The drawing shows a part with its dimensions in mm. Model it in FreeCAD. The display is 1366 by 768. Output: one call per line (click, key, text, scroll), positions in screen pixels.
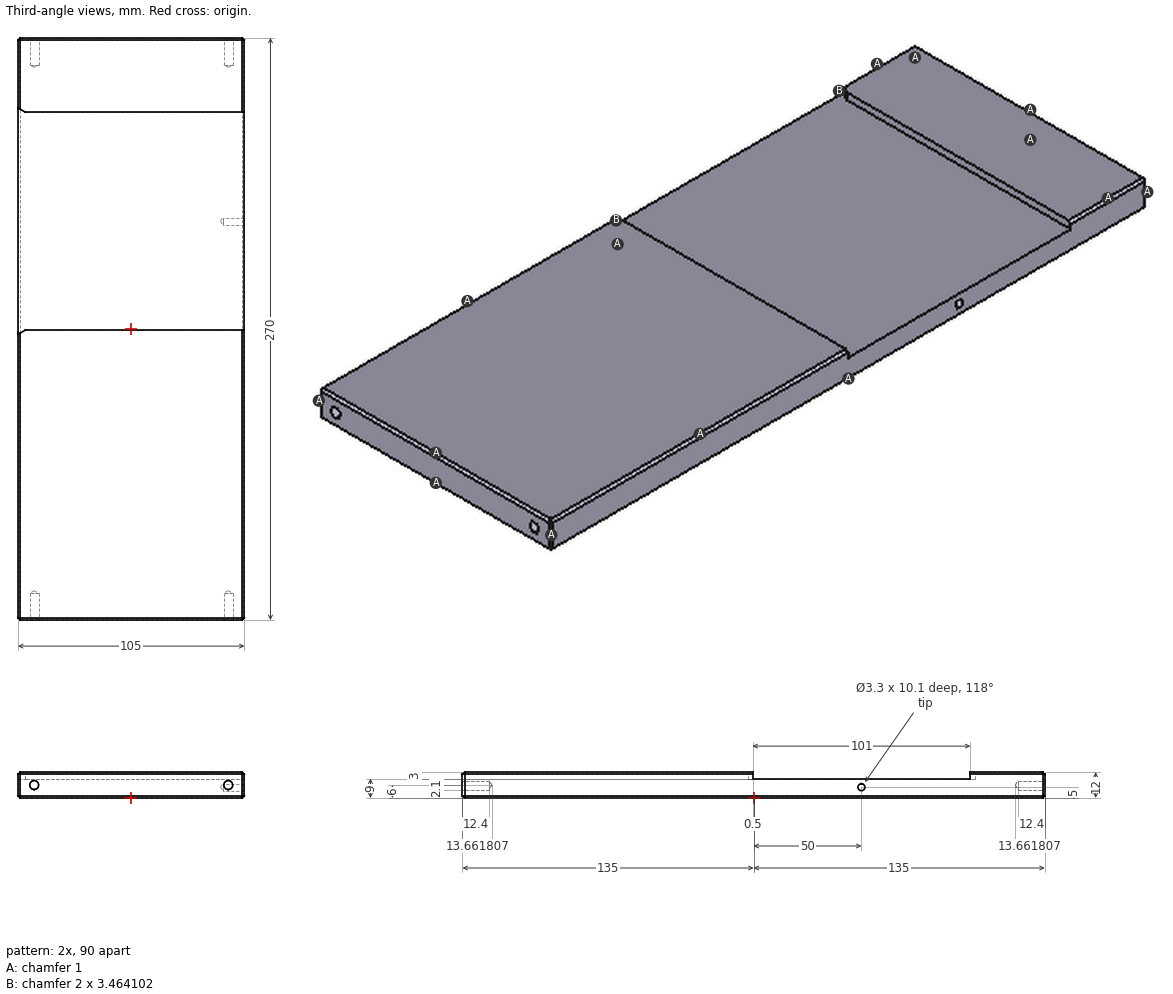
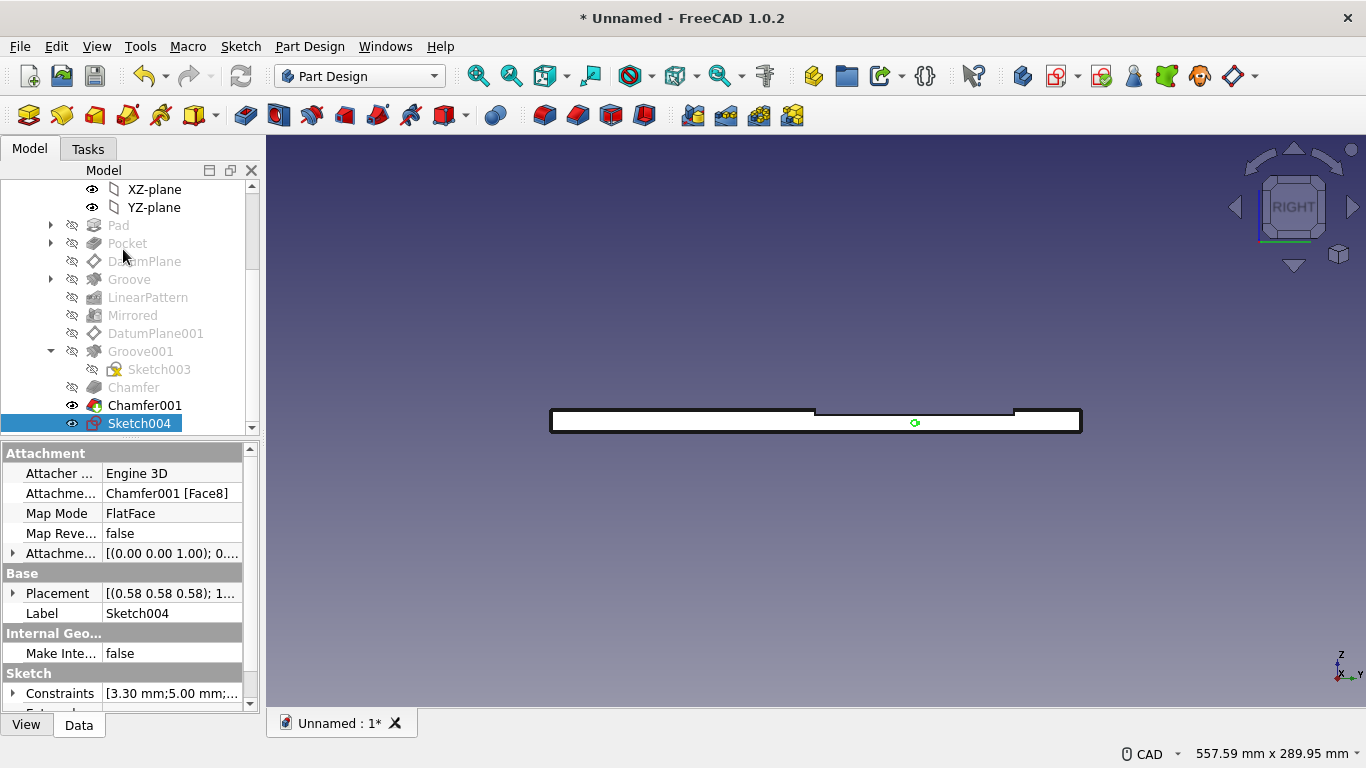
click(279, 116)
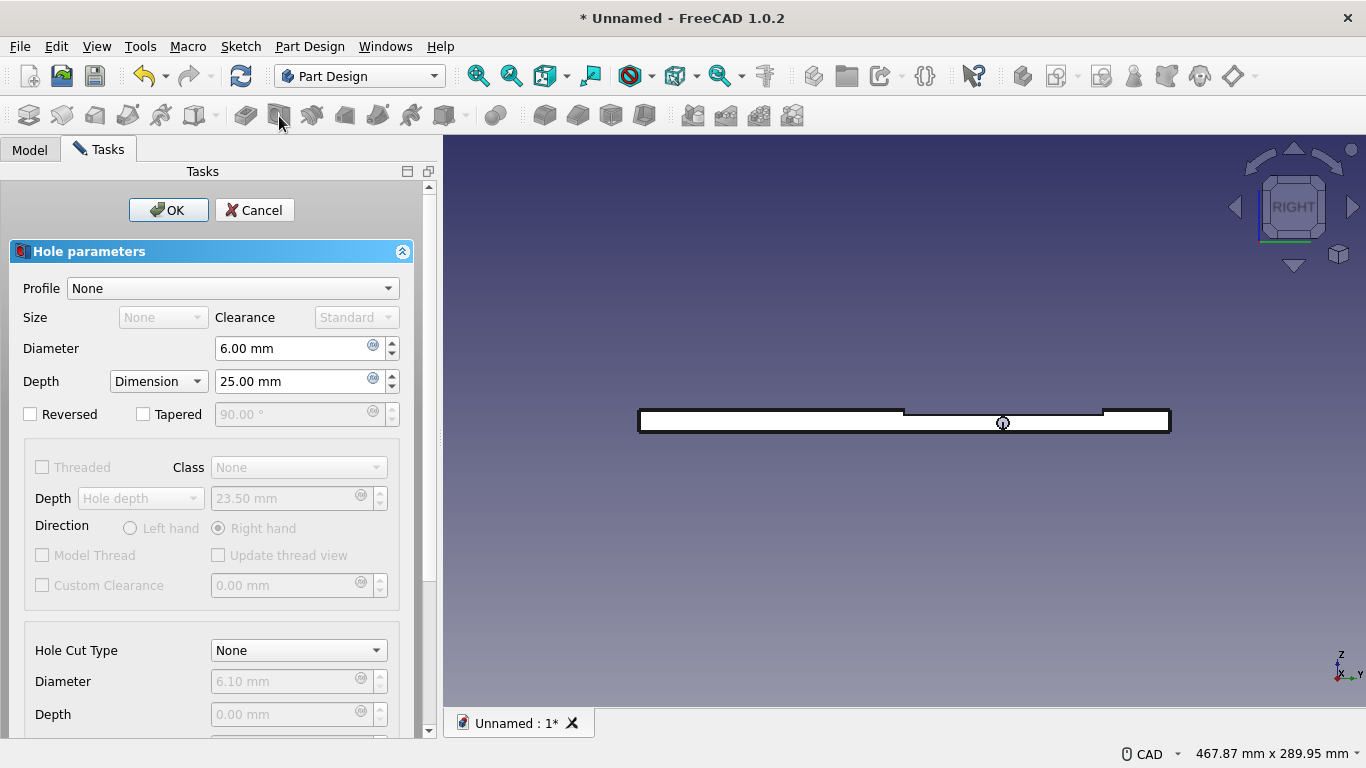
triple_click(300, 348)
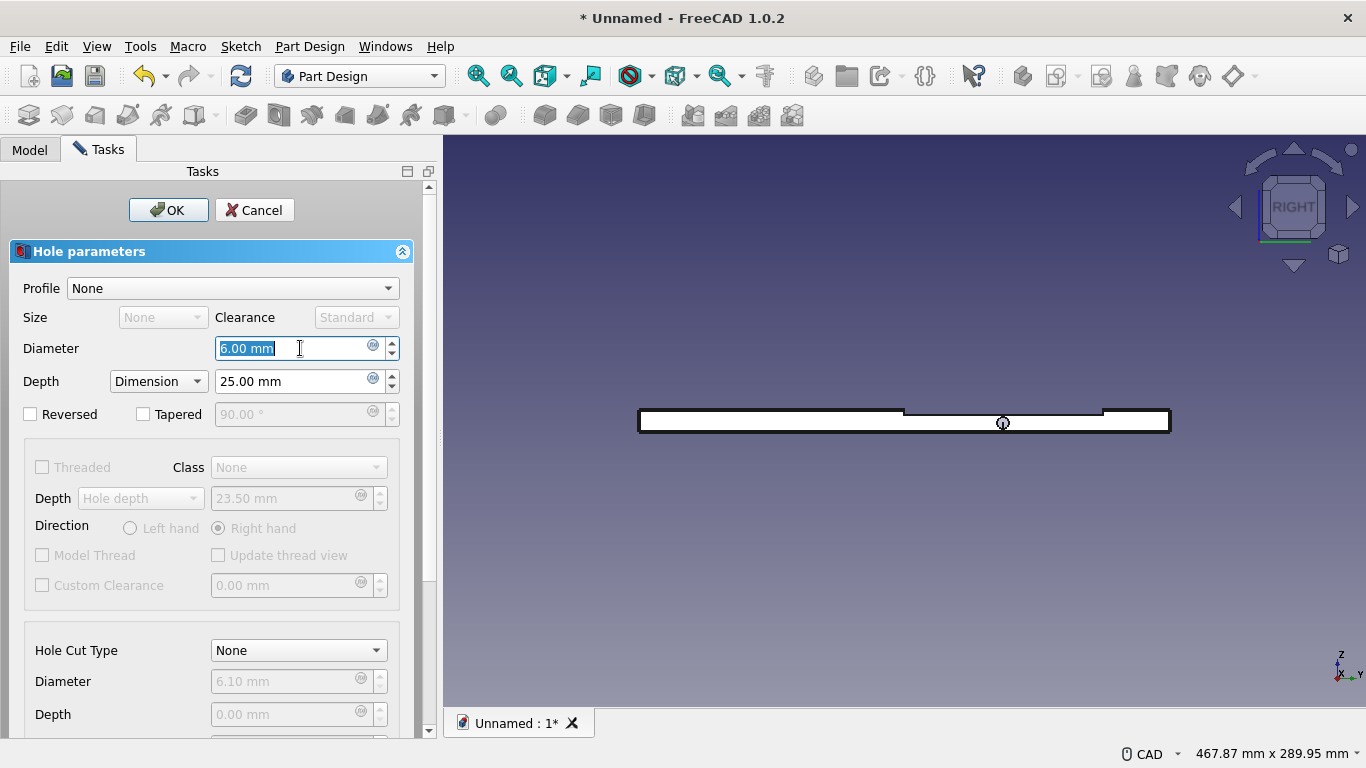
text(3.3)
key(Tab)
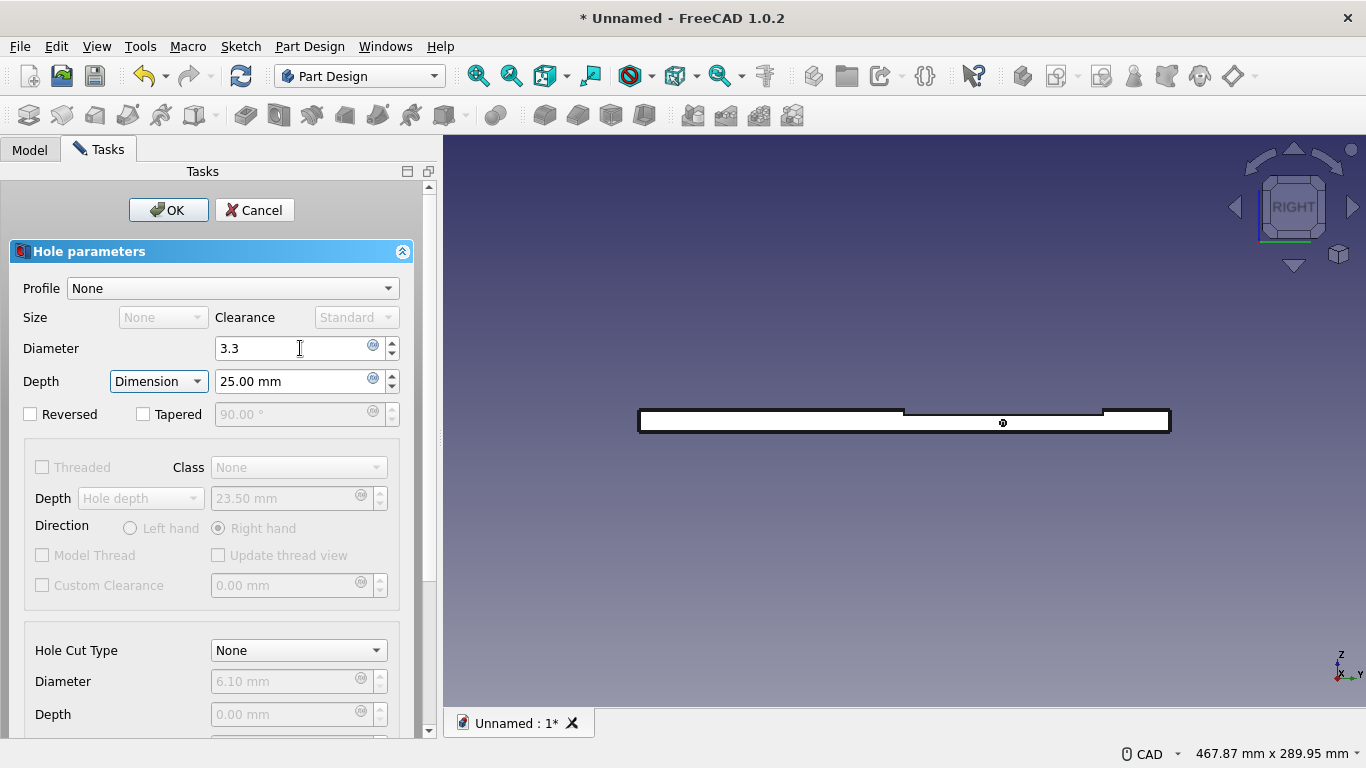
triple_click(300, 382)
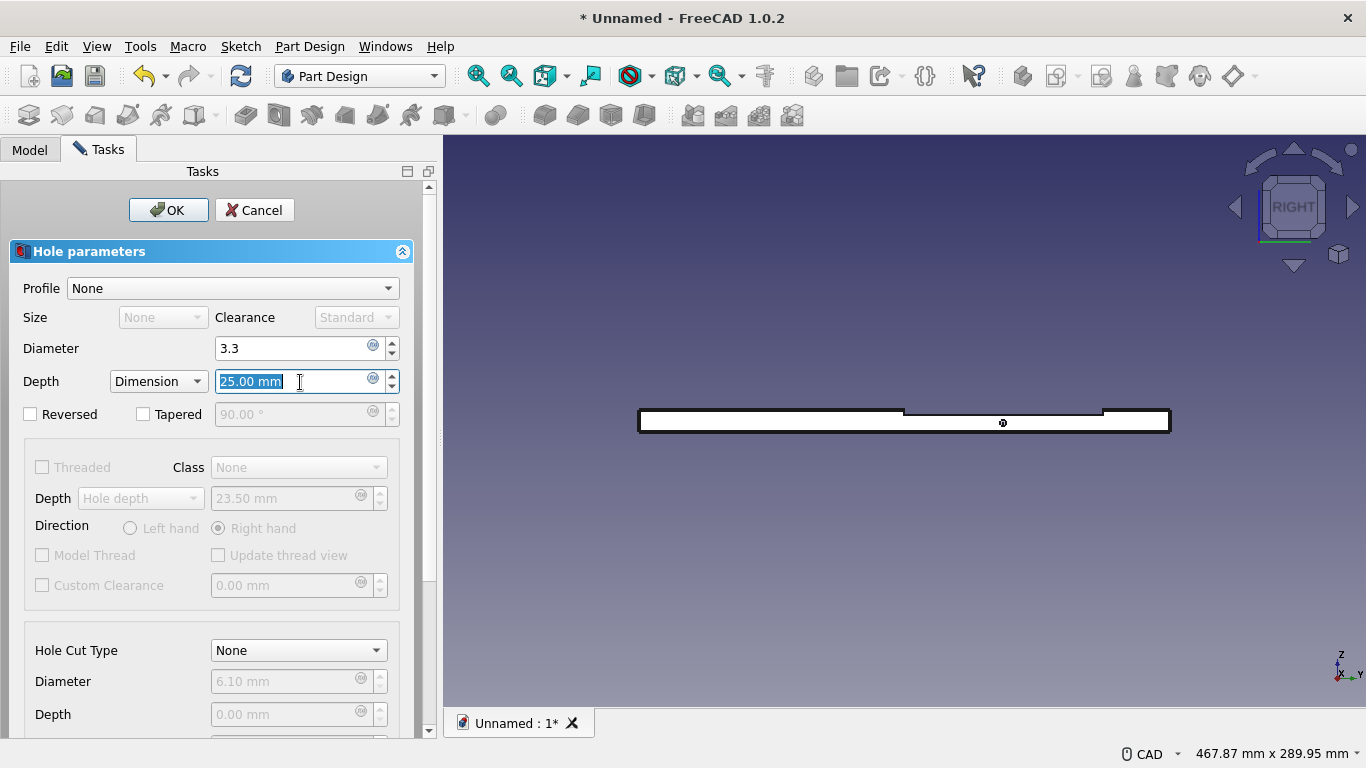
text(10.1)
key(Tab)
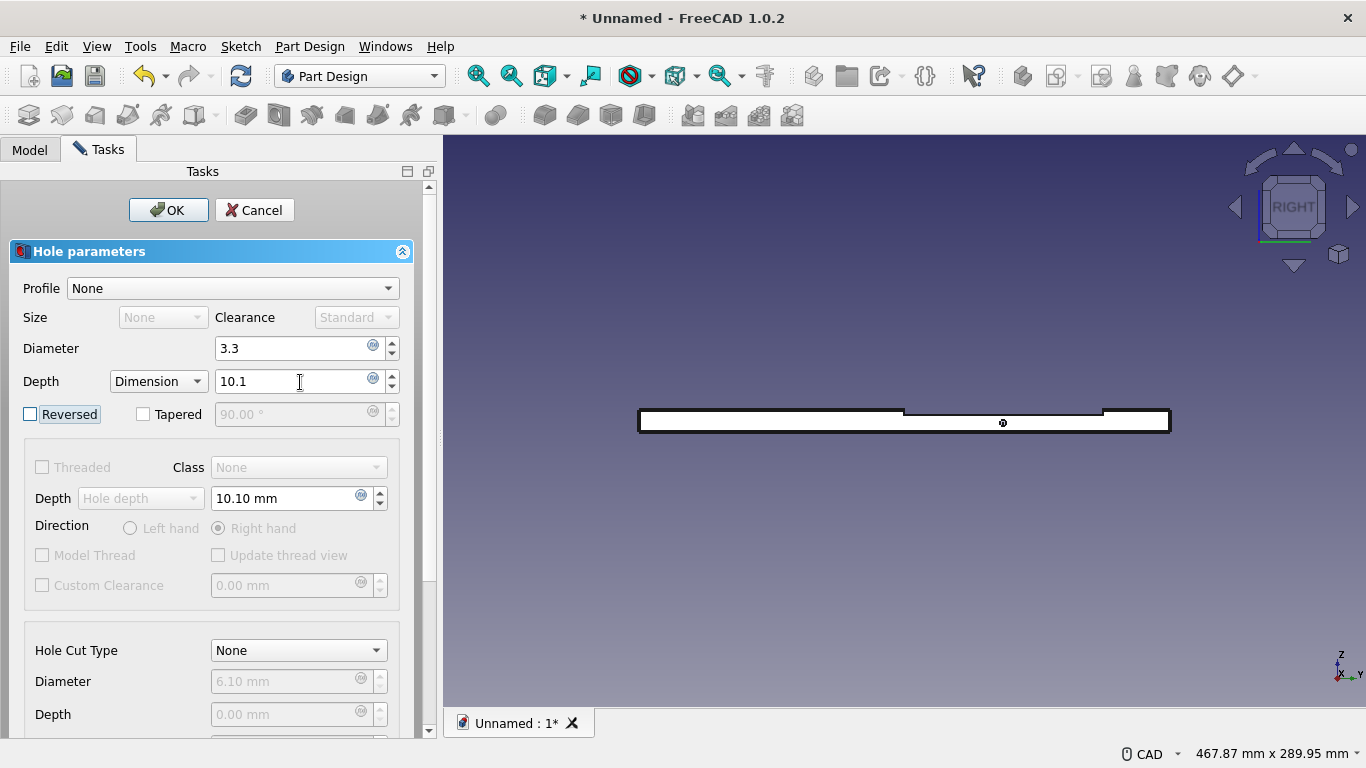
click(169, 210)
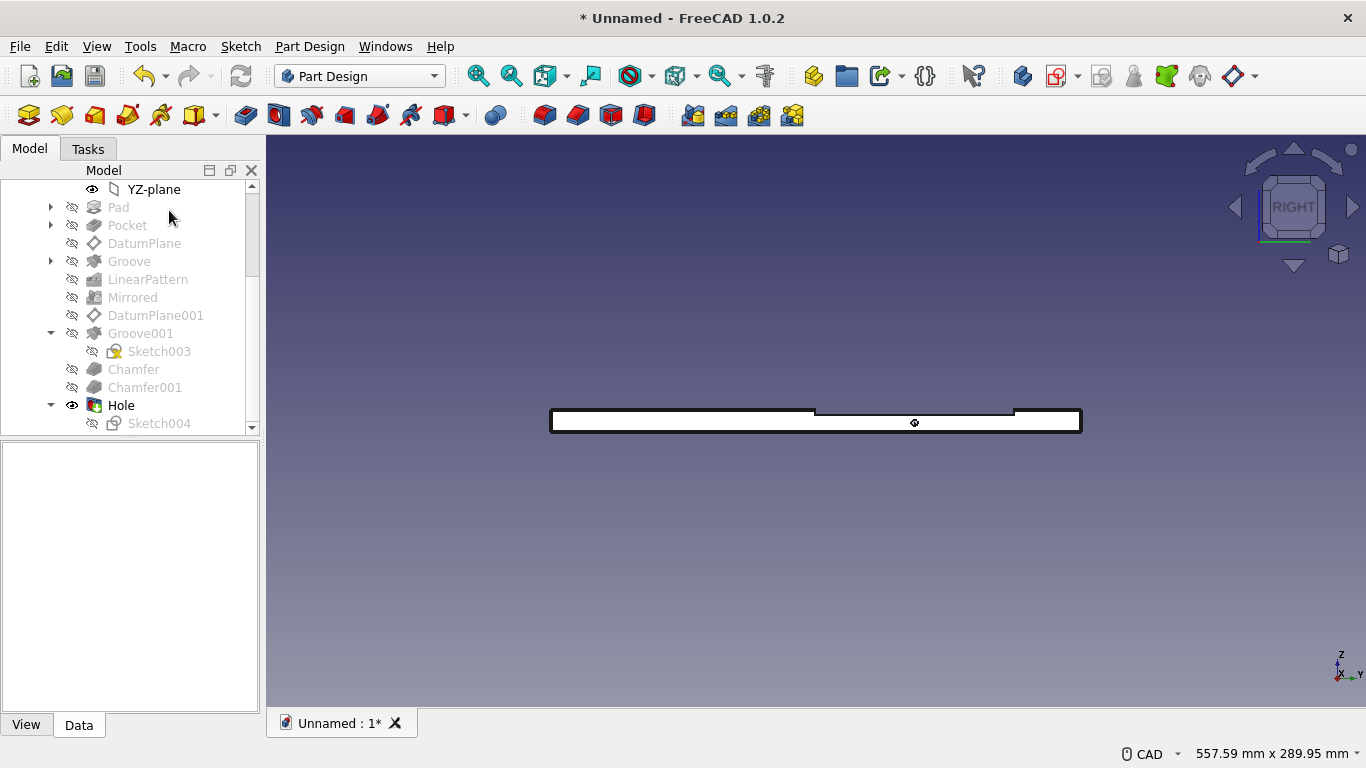
key(0)